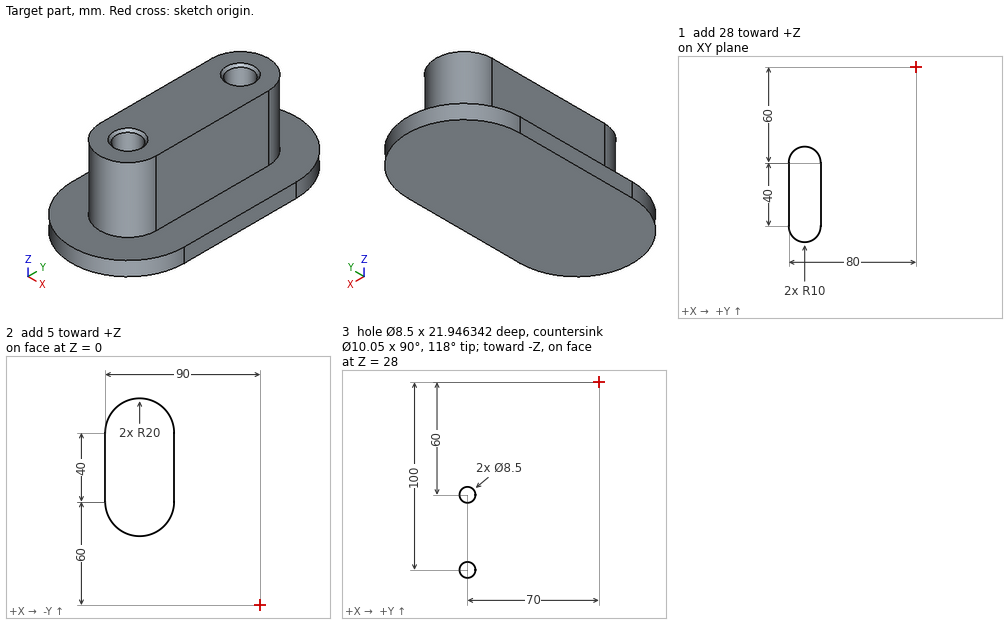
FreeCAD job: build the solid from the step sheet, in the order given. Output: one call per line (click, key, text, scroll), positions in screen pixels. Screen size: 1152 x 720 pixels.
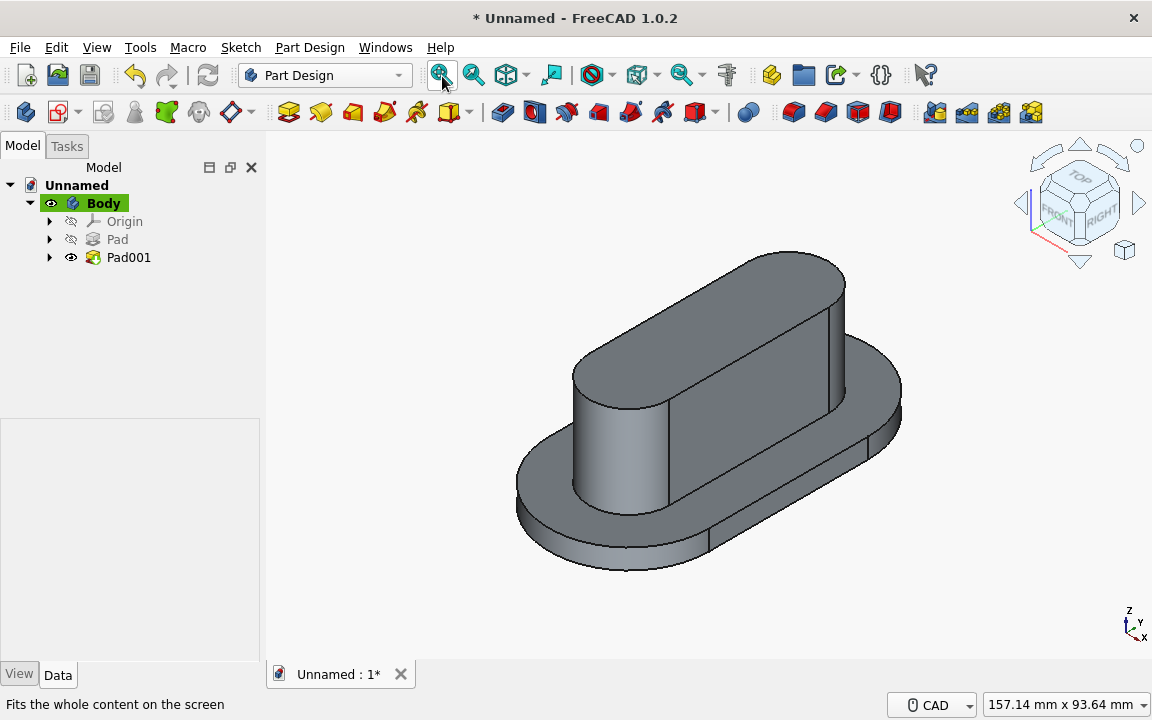
click(777, 290)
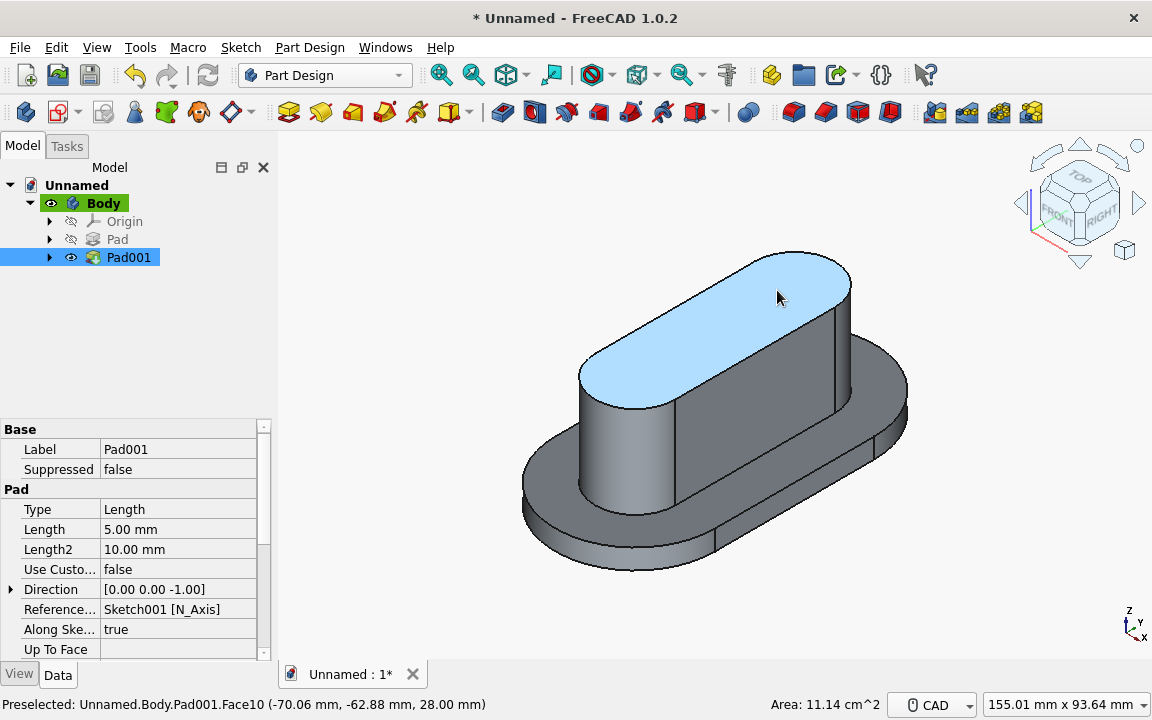
click(58, 112)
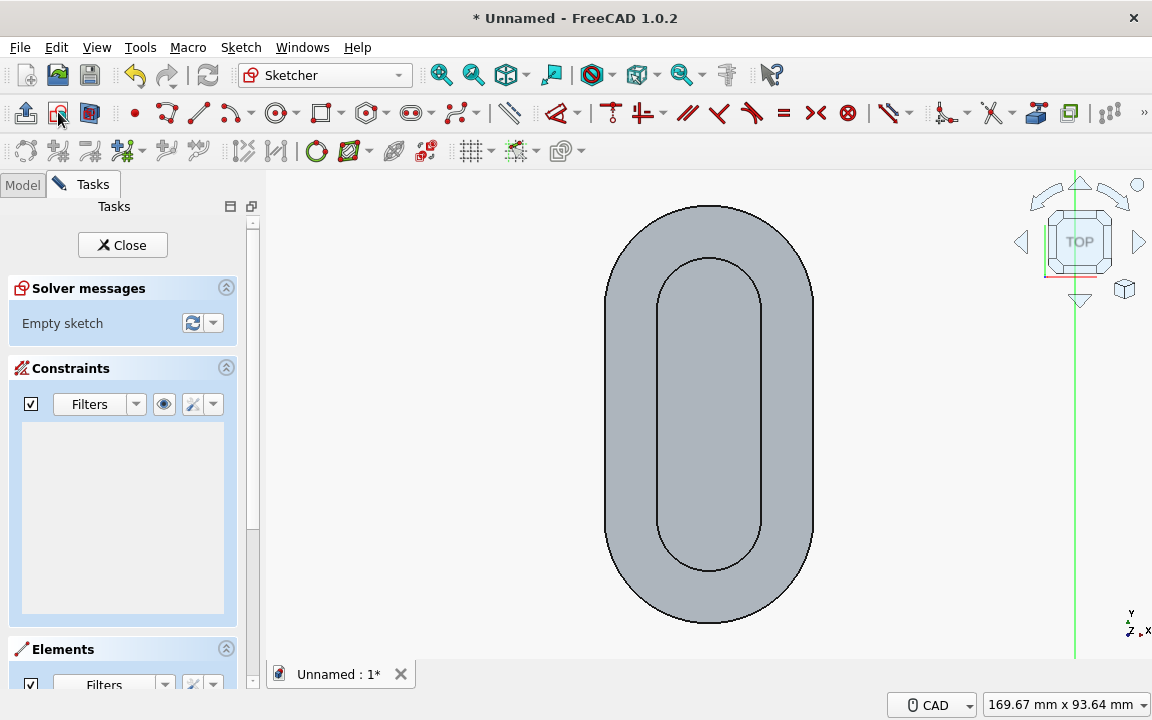
scroll(348, 592, down, 3)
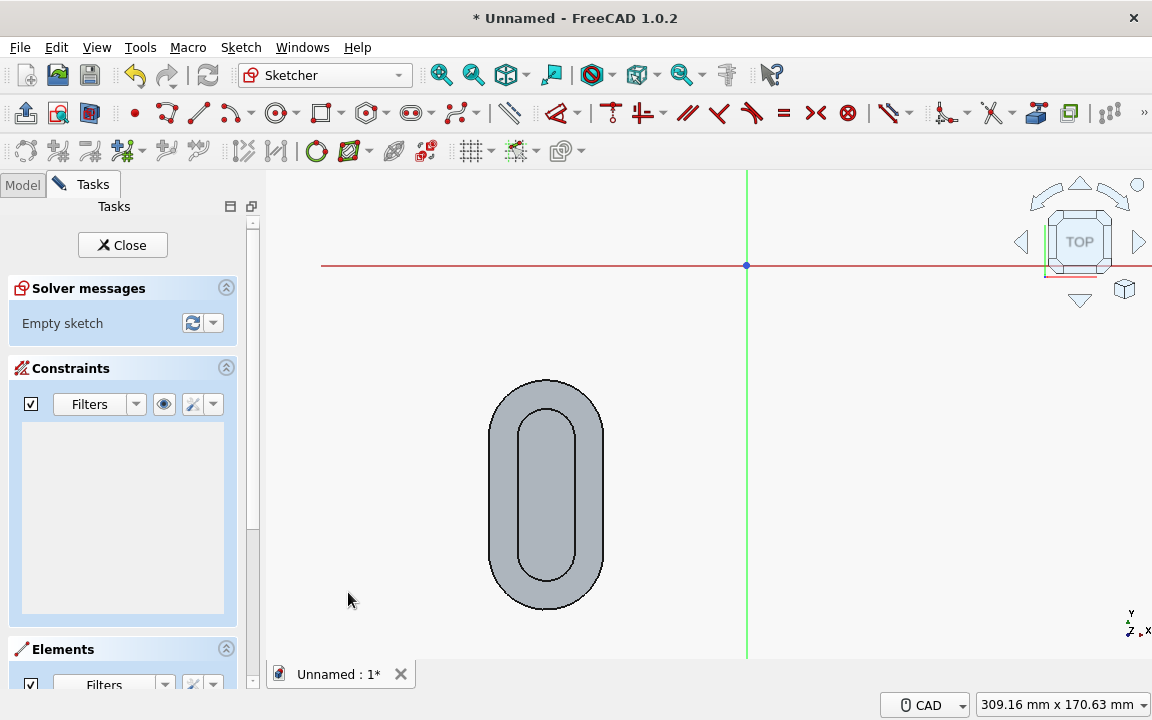
click(276, 114)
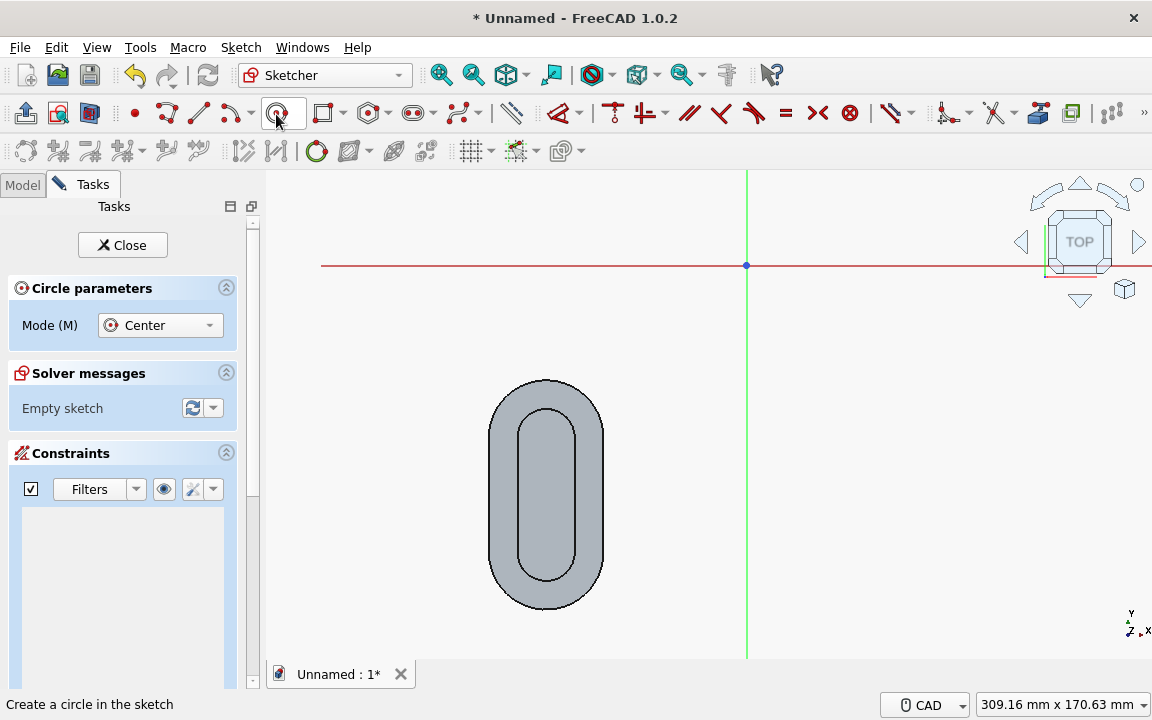
scroll(546, 438, up, 4)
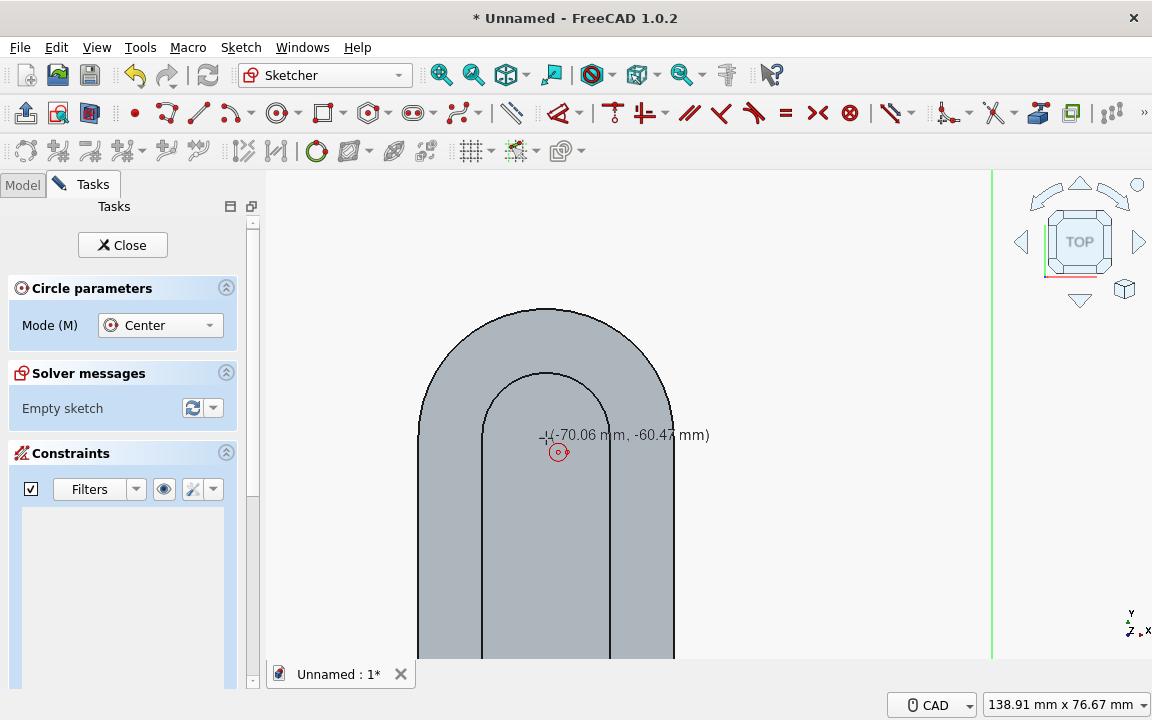
click(546, 437)
click(565, 417)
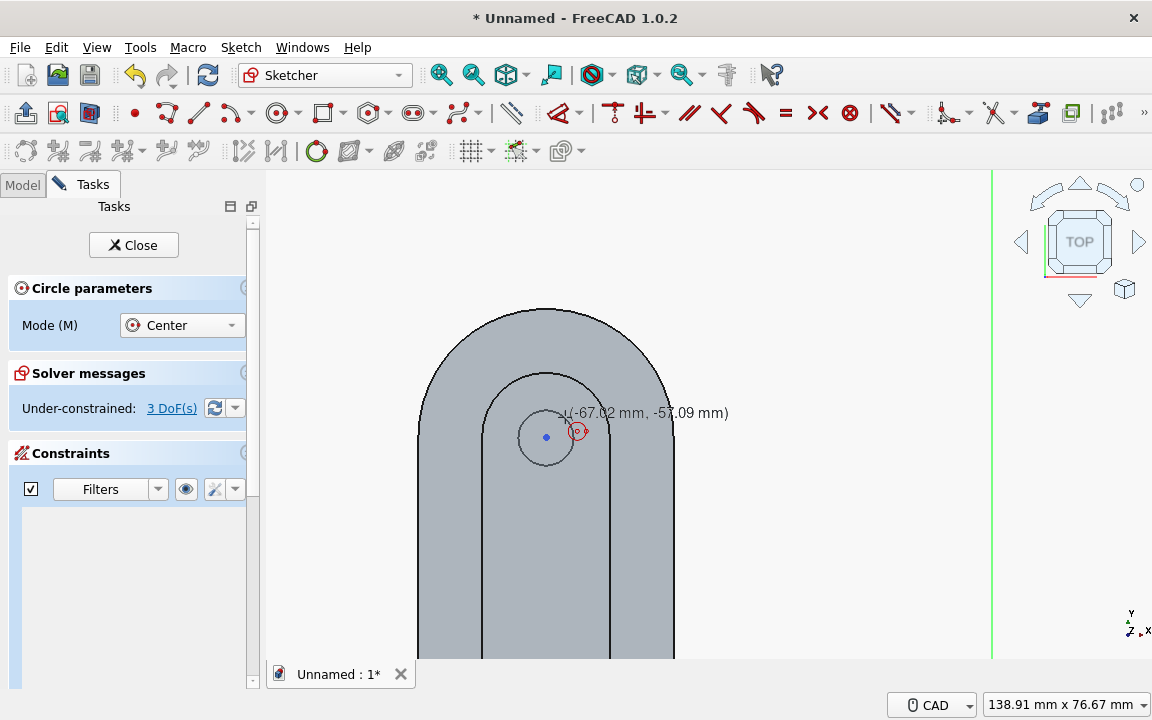
scroll(547, 437, down, 4)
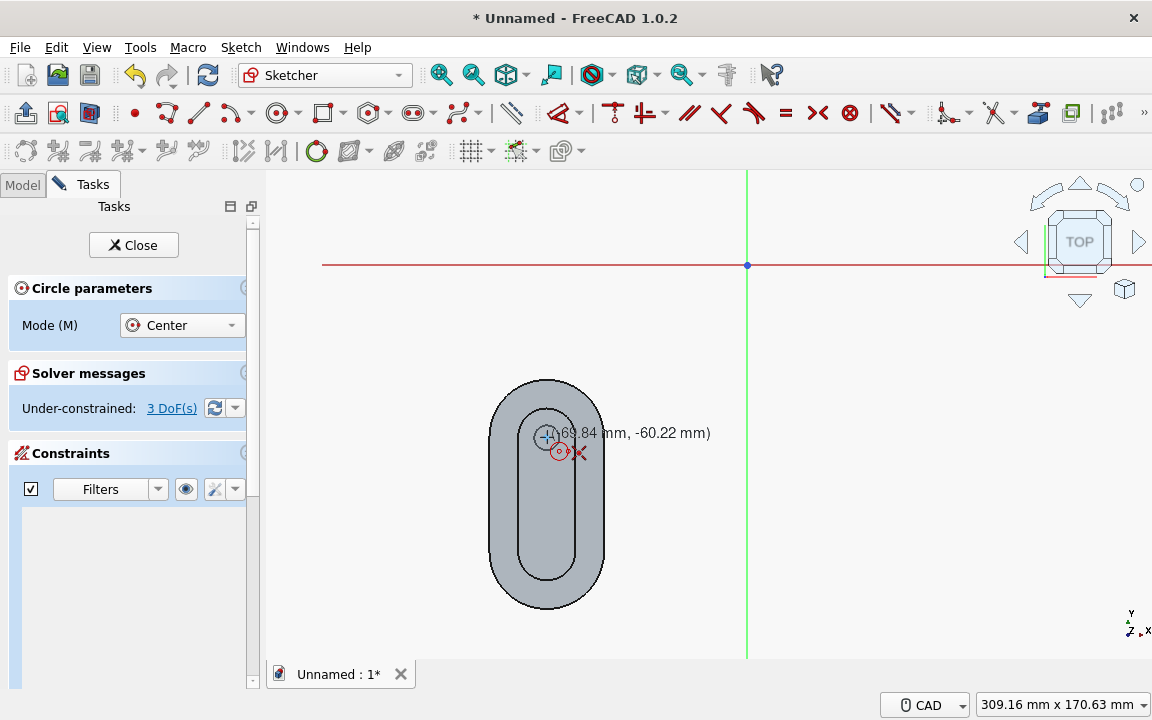
scroll(547, 552, up, 4)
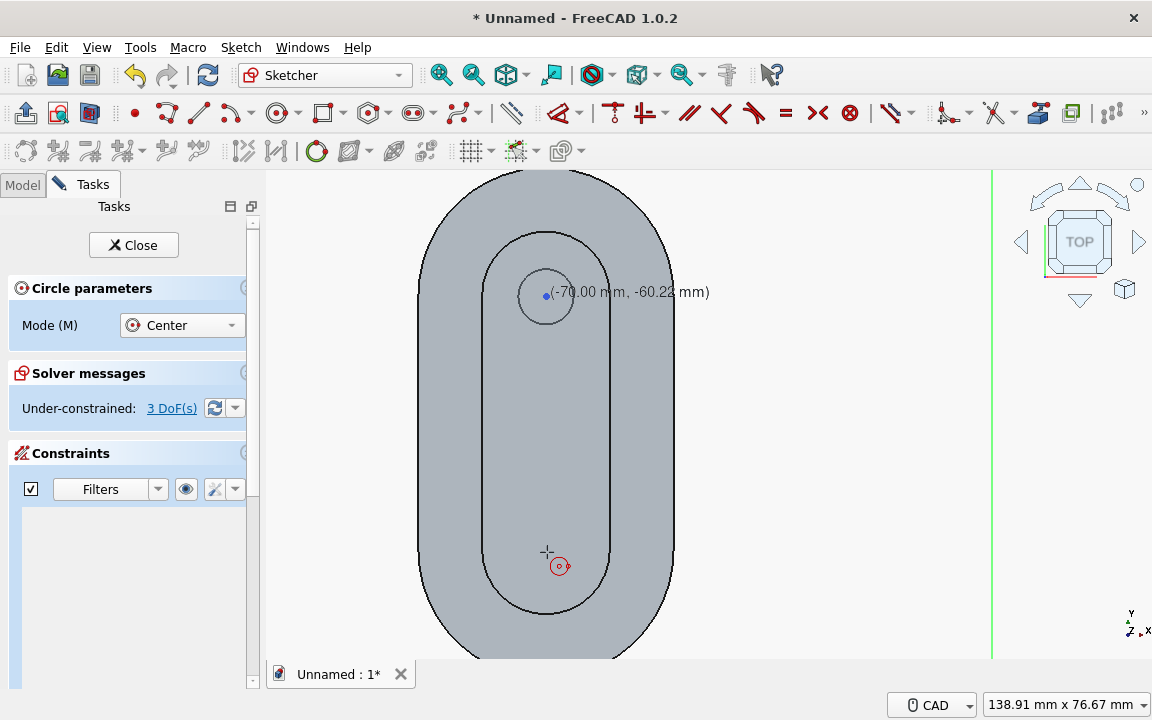
click(546, 550)
click(565, 531)
key(Escape)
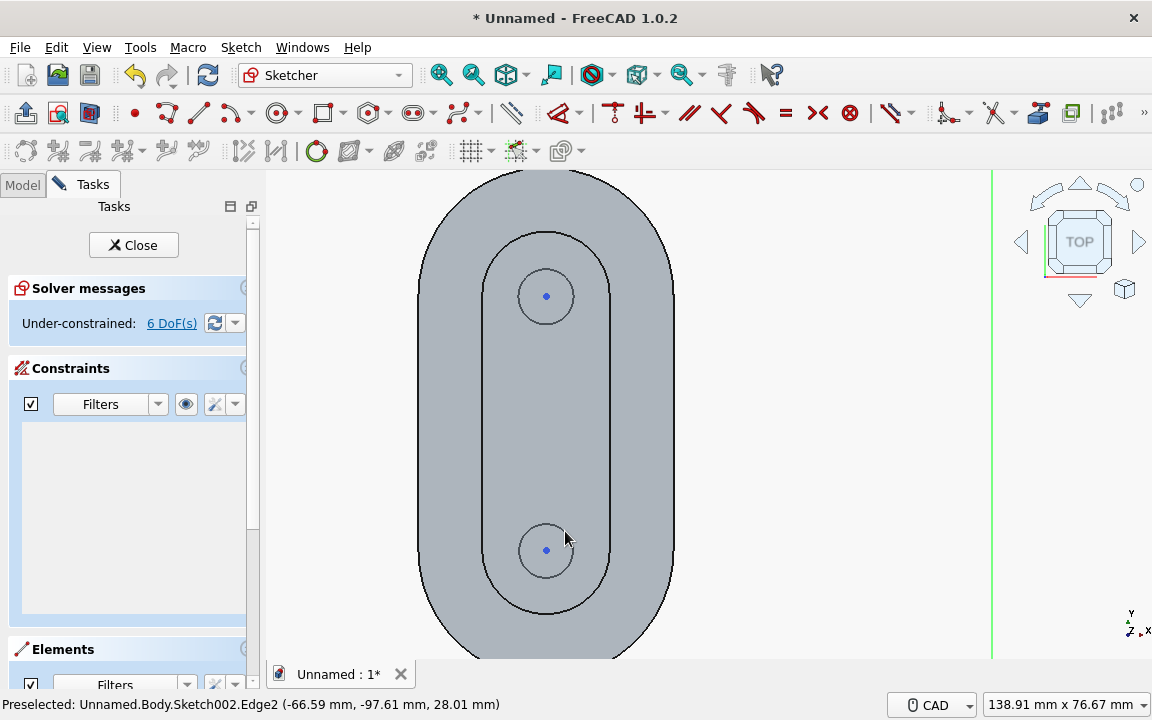
click(565, 277)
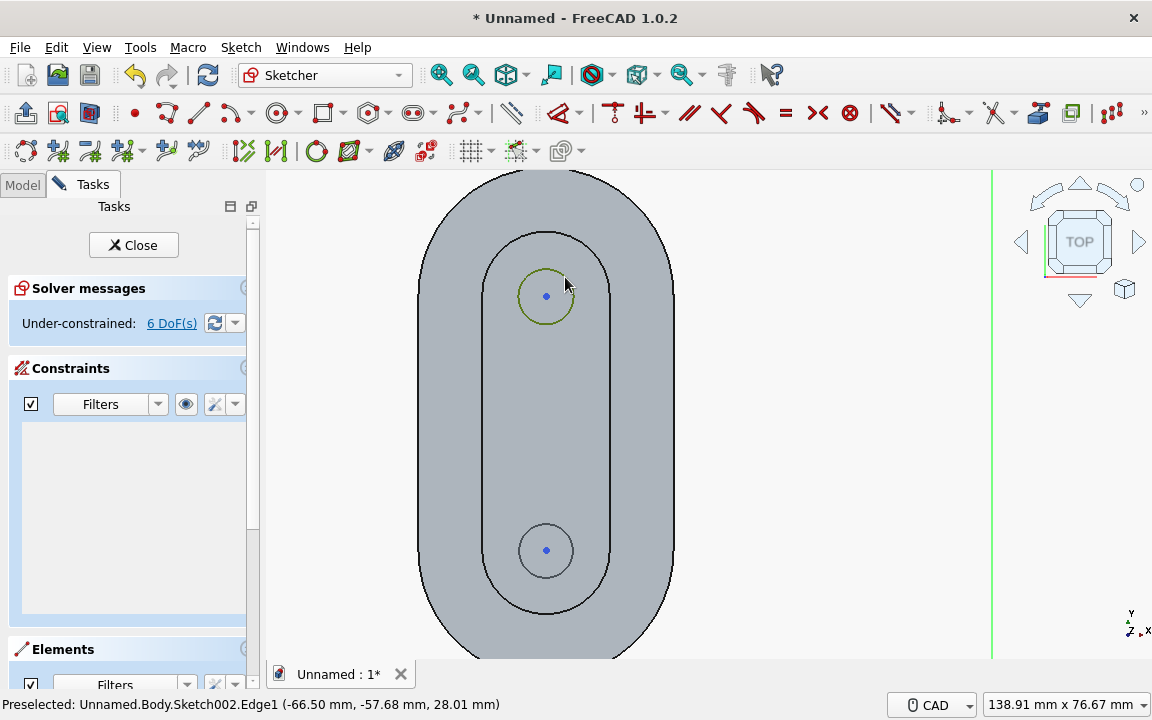
click(565, 532)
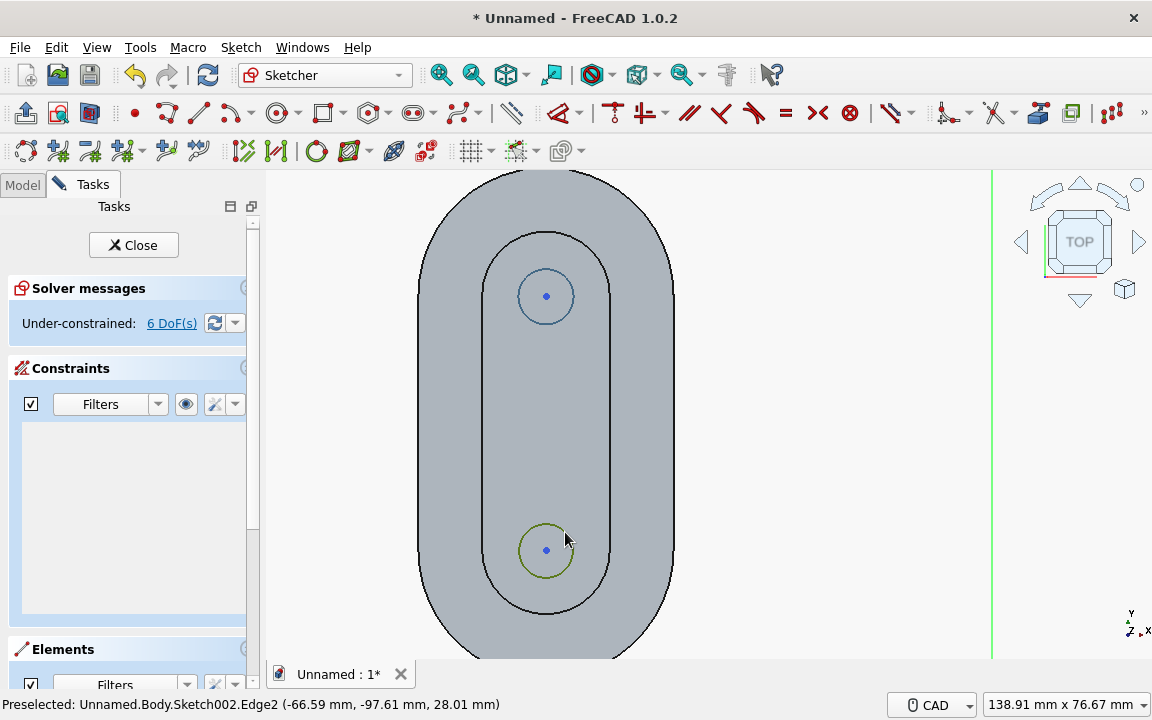
click(786, 114)